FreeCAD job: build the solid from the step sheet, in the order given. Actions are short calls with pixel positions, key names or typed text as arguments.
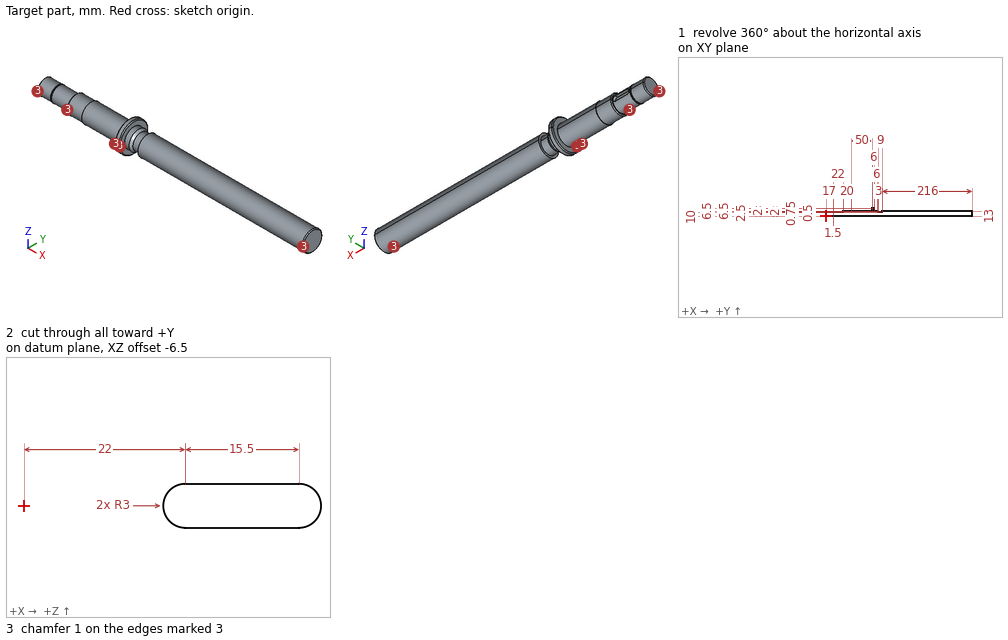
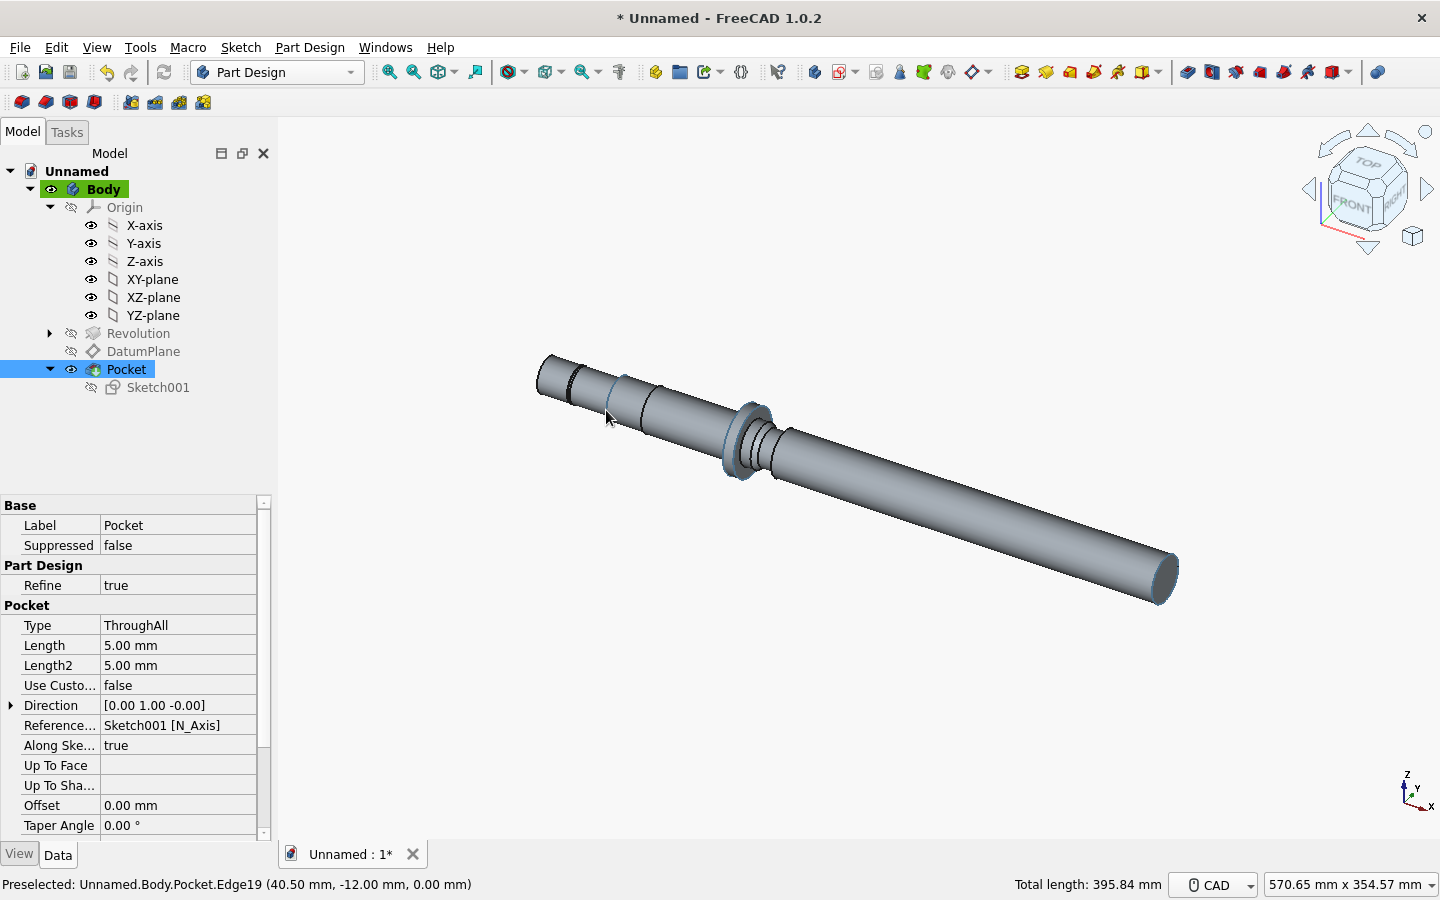
click(537, 384, ctrl)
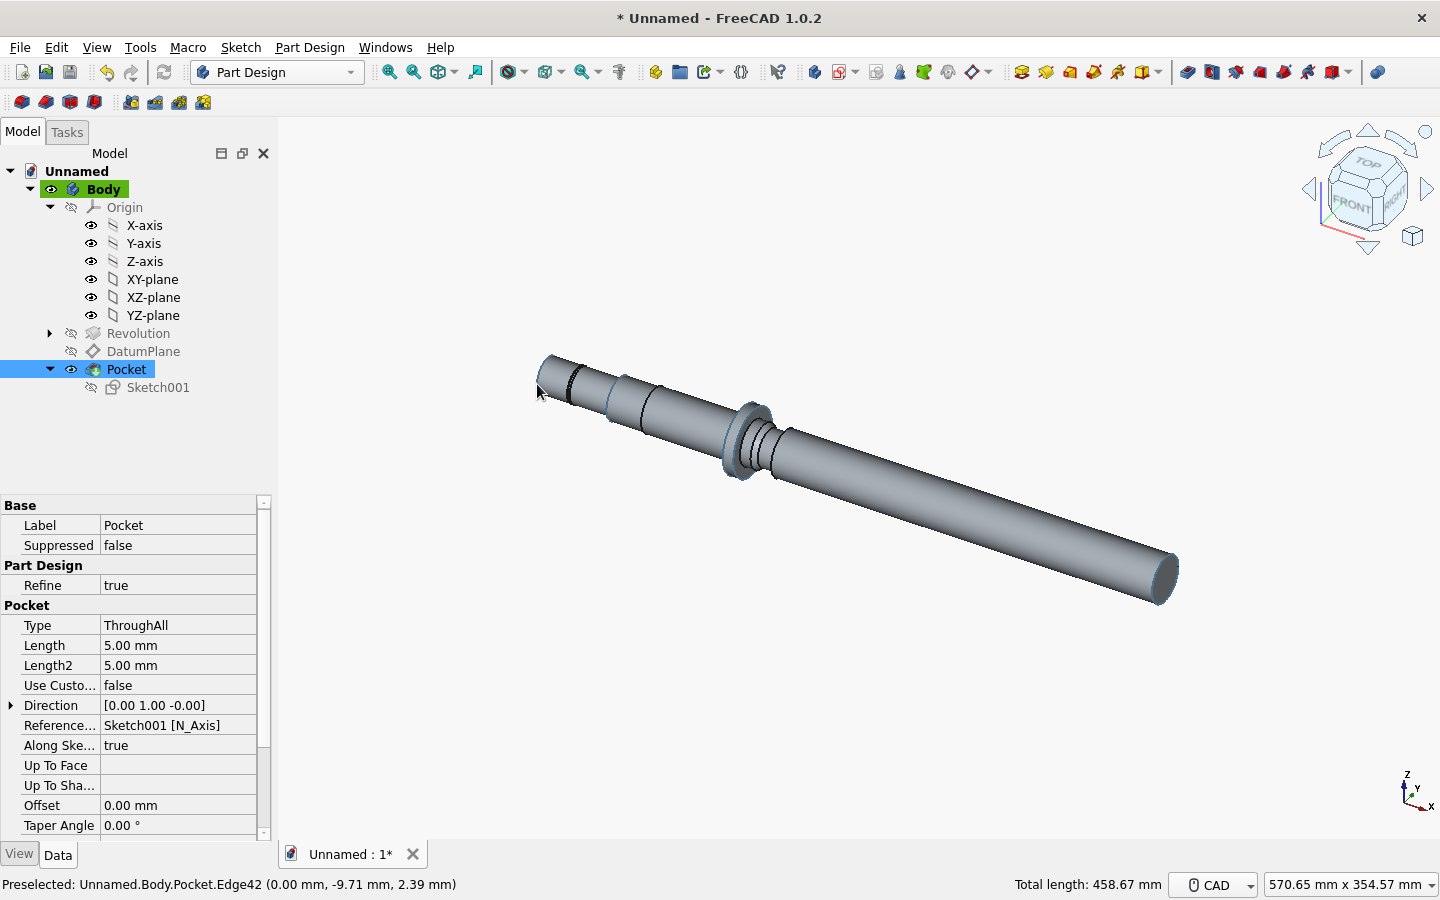
click(46, 102)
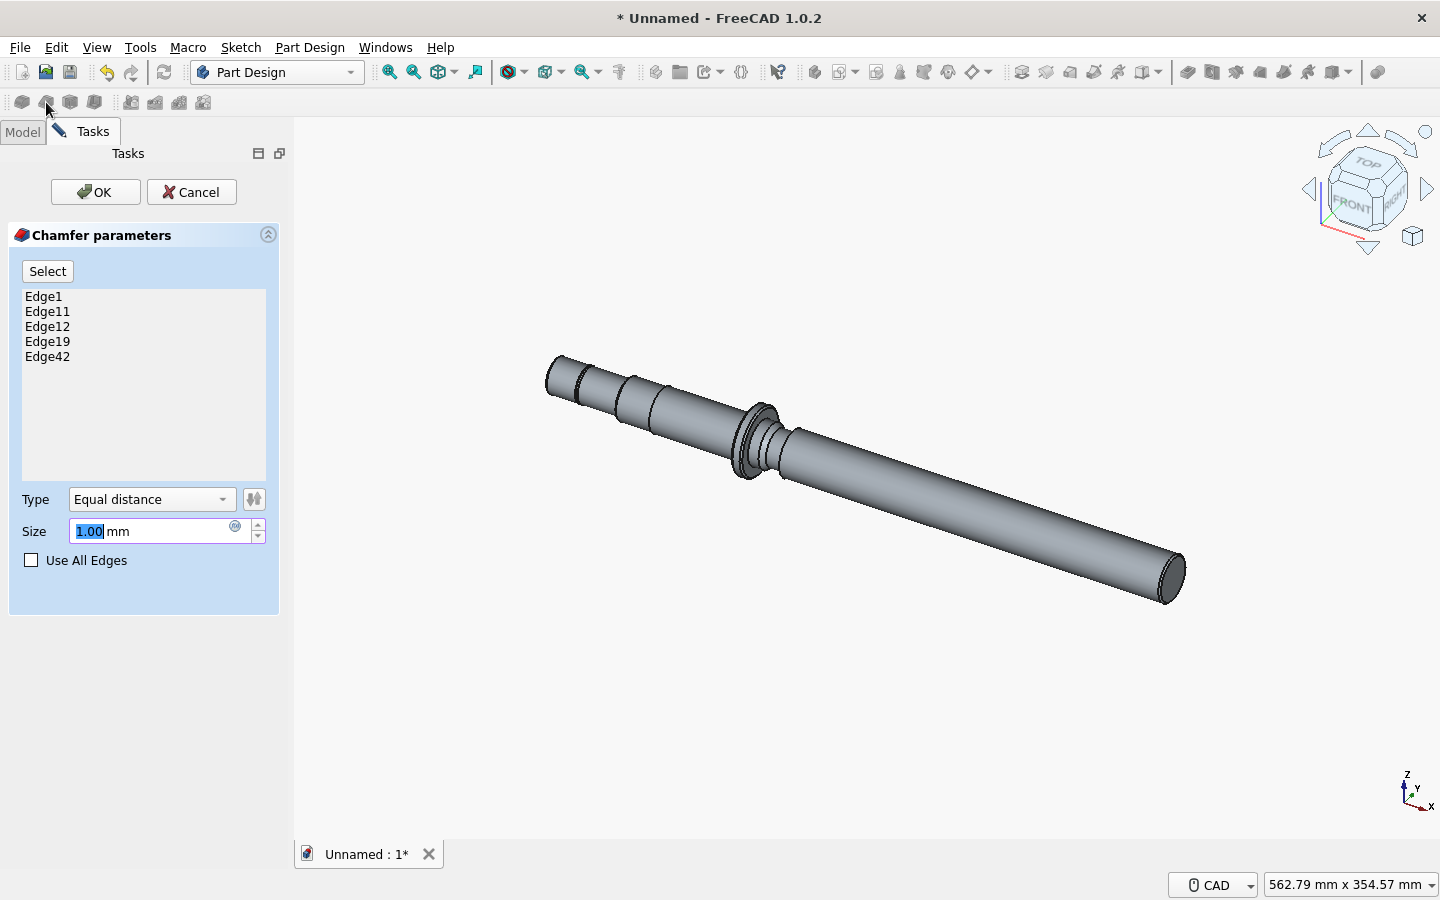
text(1)
key(Tab)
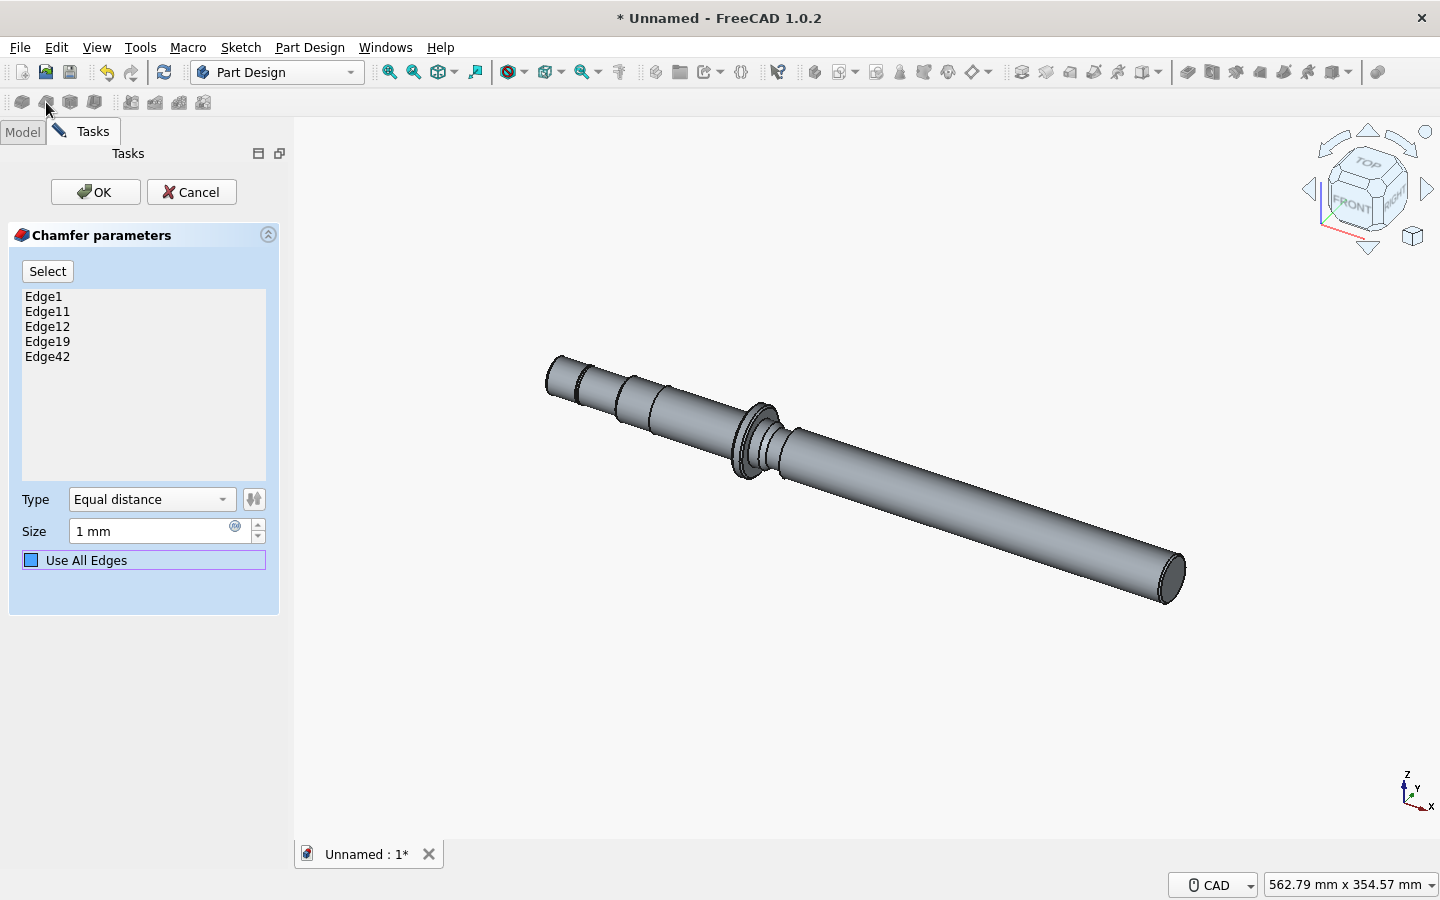
click(96, 192)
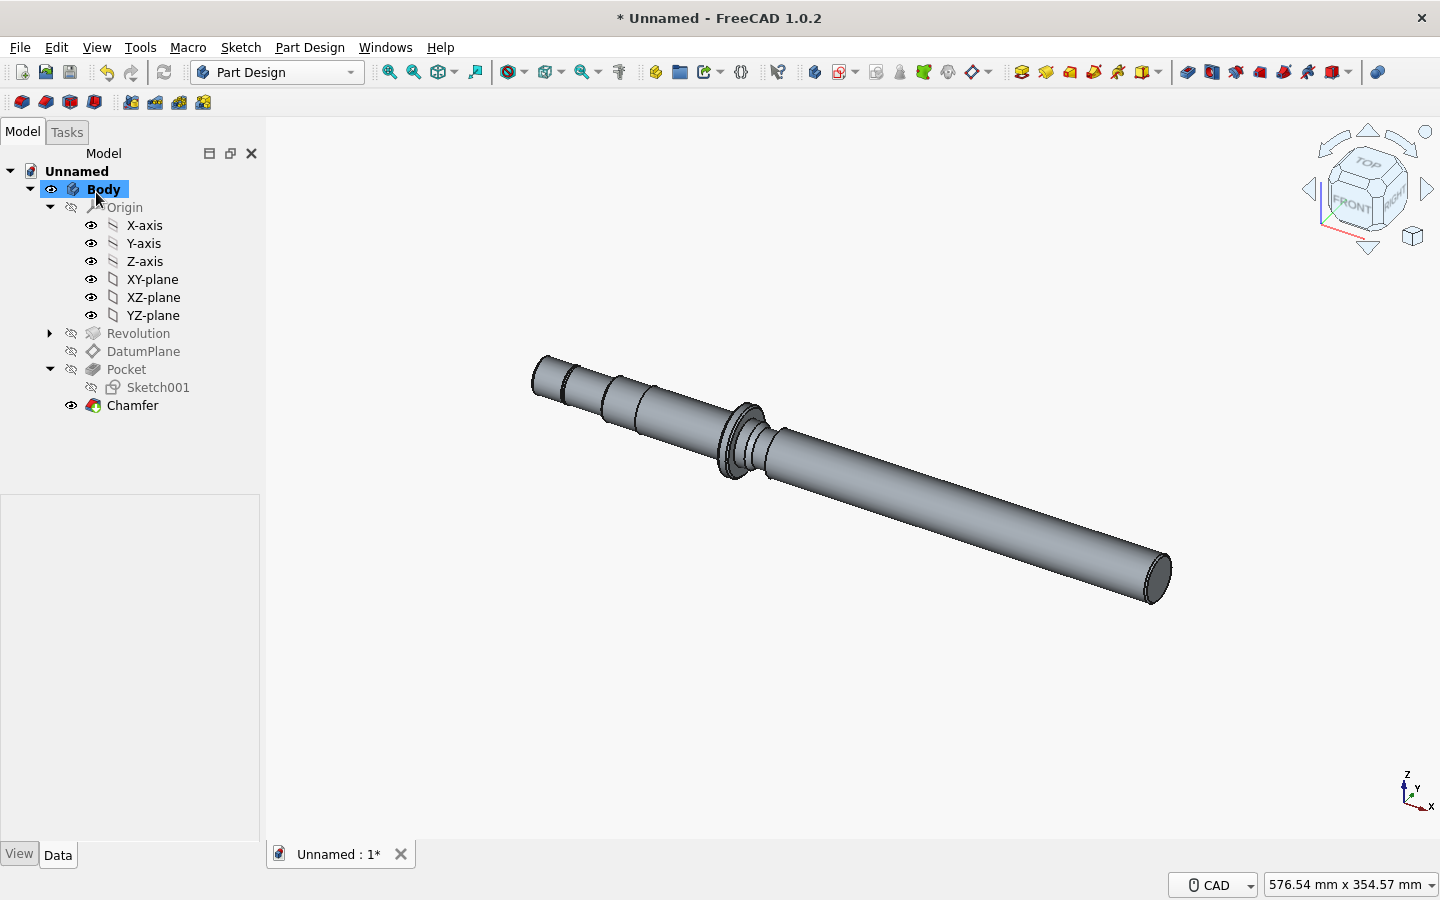
key(0)